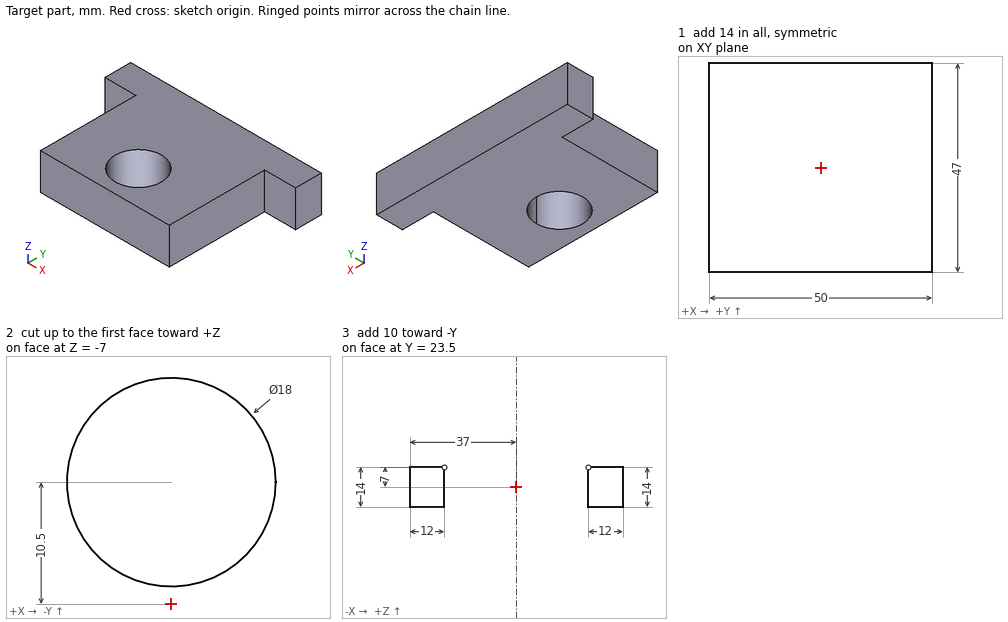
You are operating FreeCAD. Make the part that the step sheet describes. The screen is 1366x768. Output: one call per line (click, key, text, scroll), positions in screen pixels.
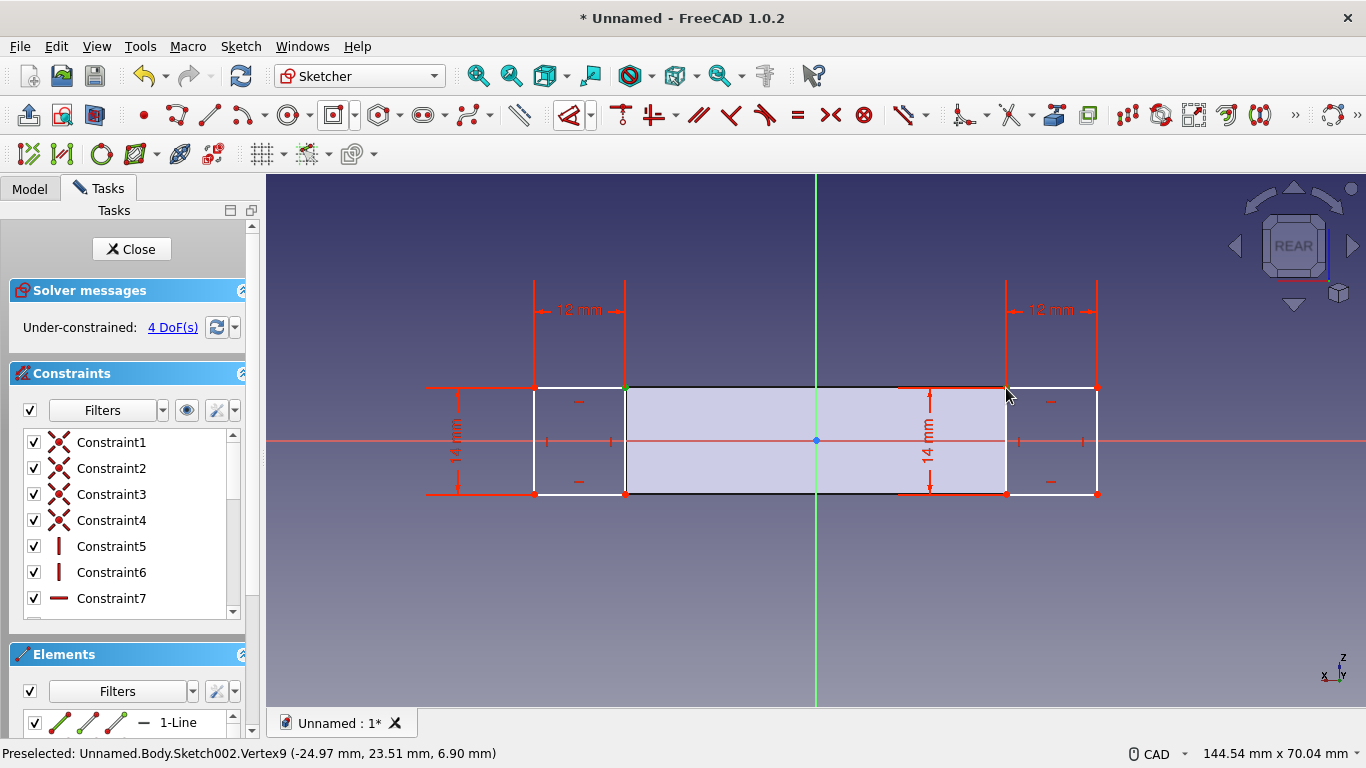
click(816, 645)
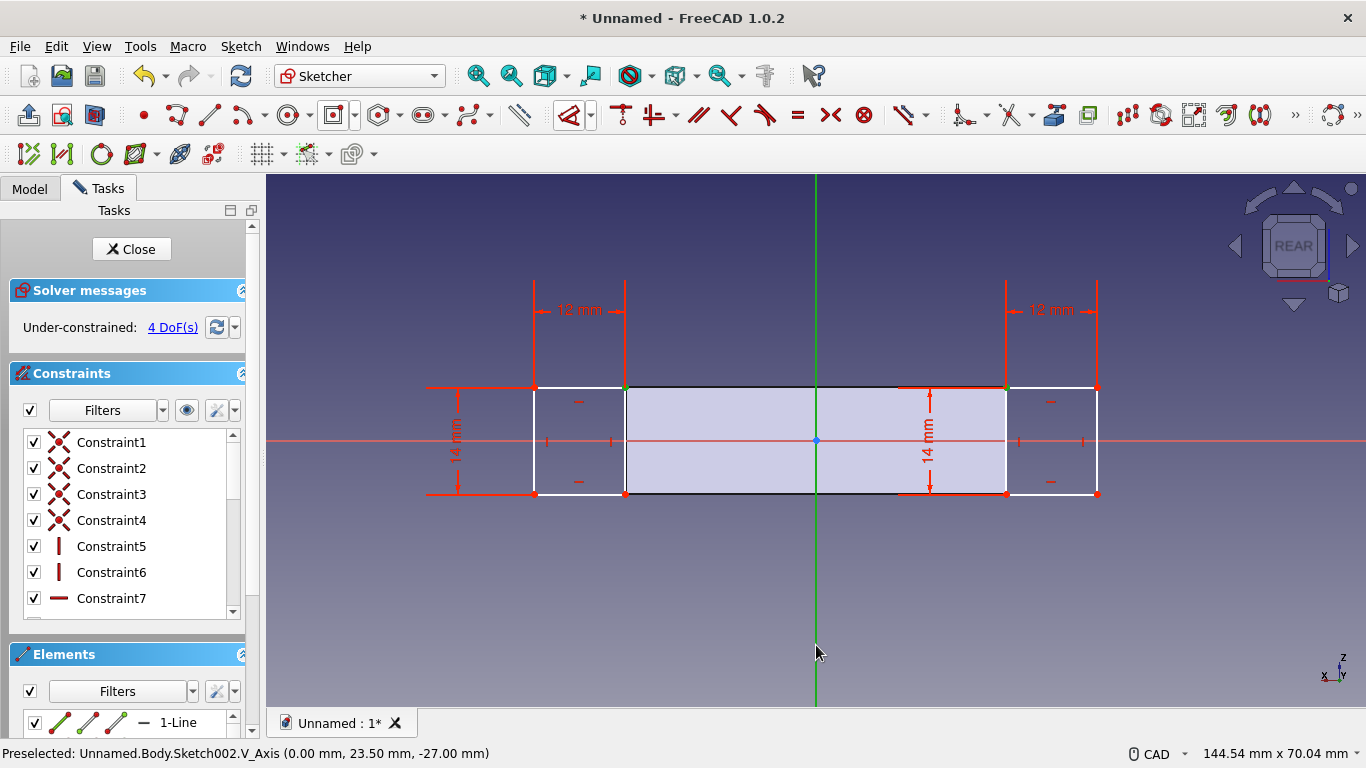
click(831, 116)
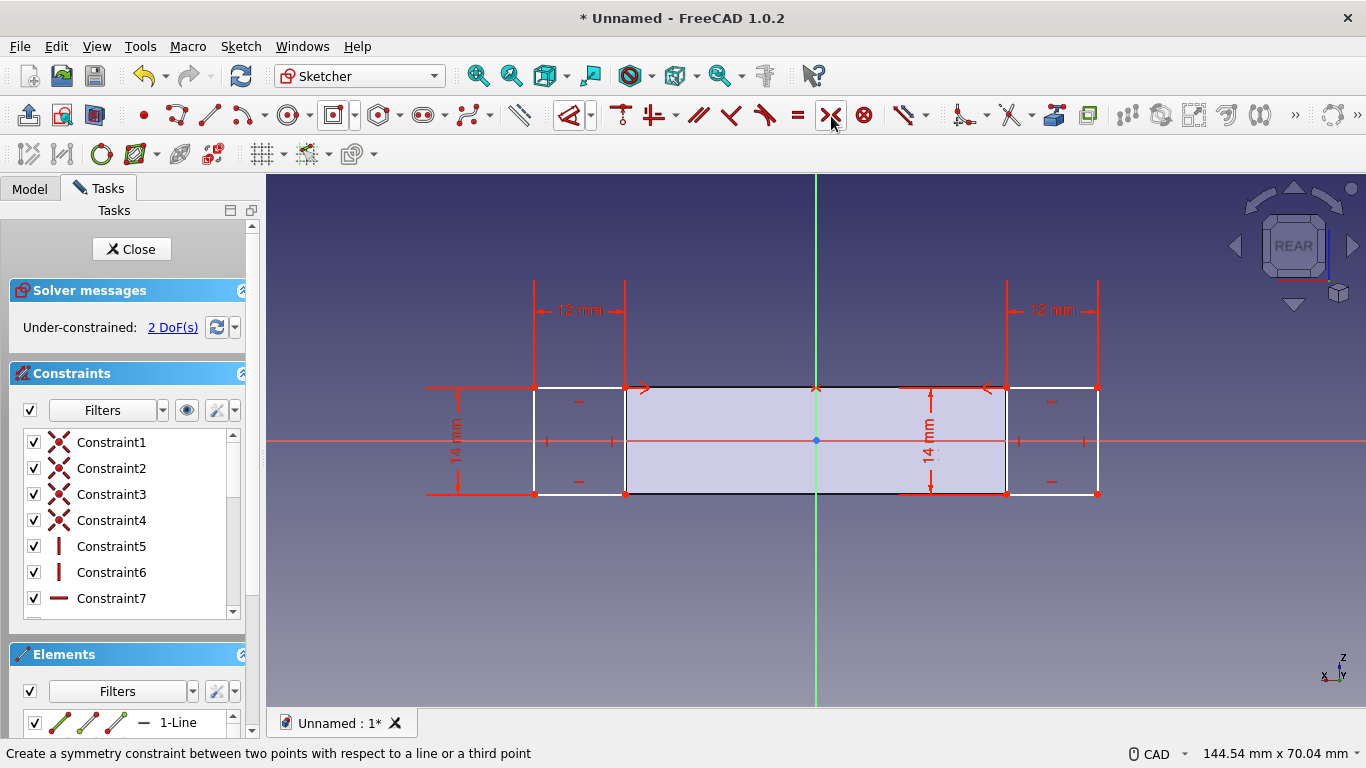
click(534, 388)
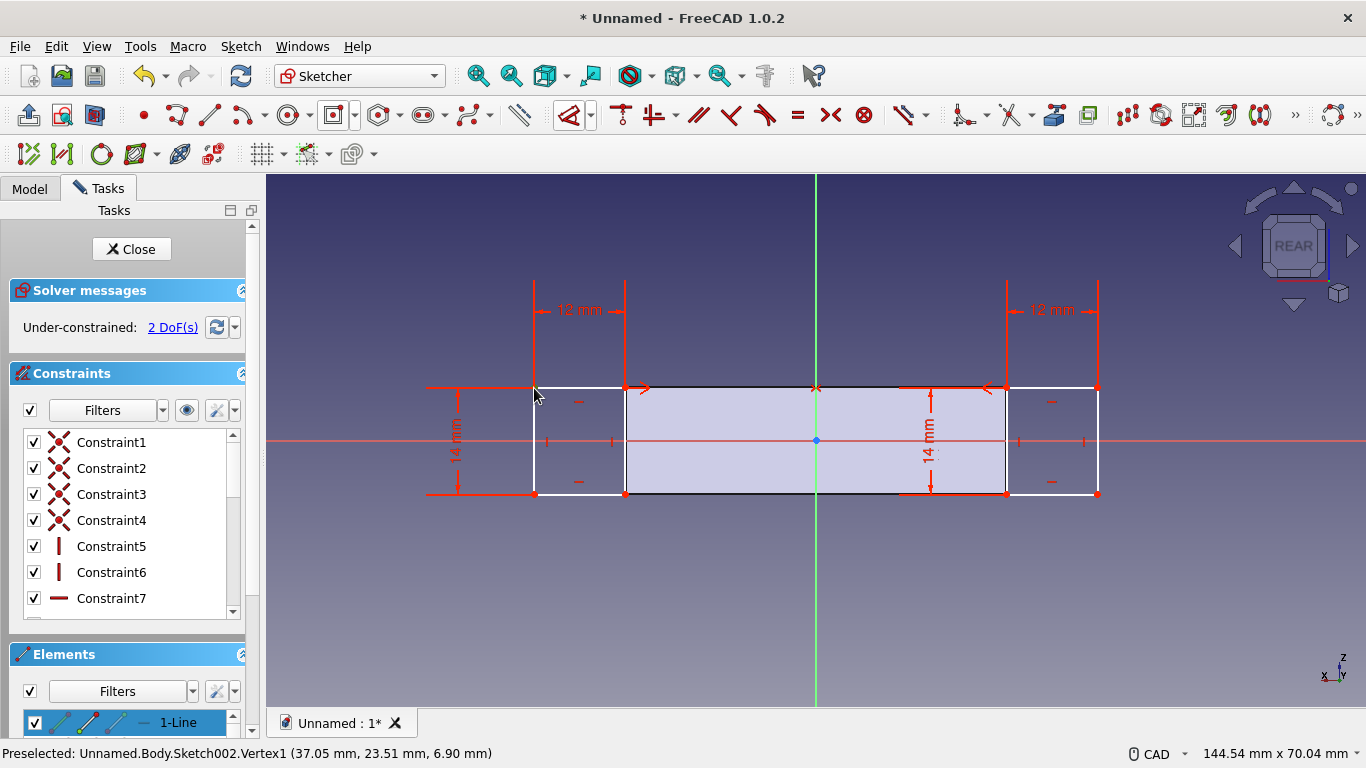
click(590, 116)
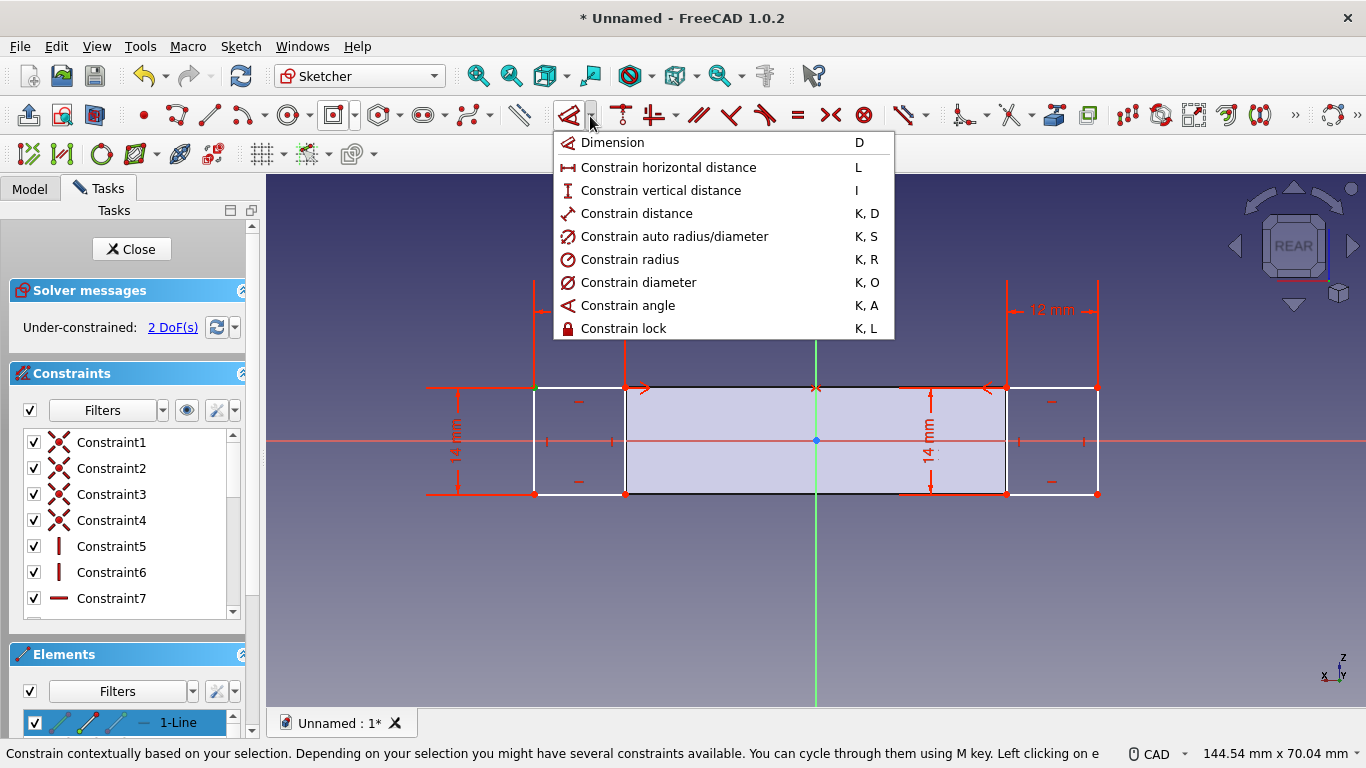
click(724, 190)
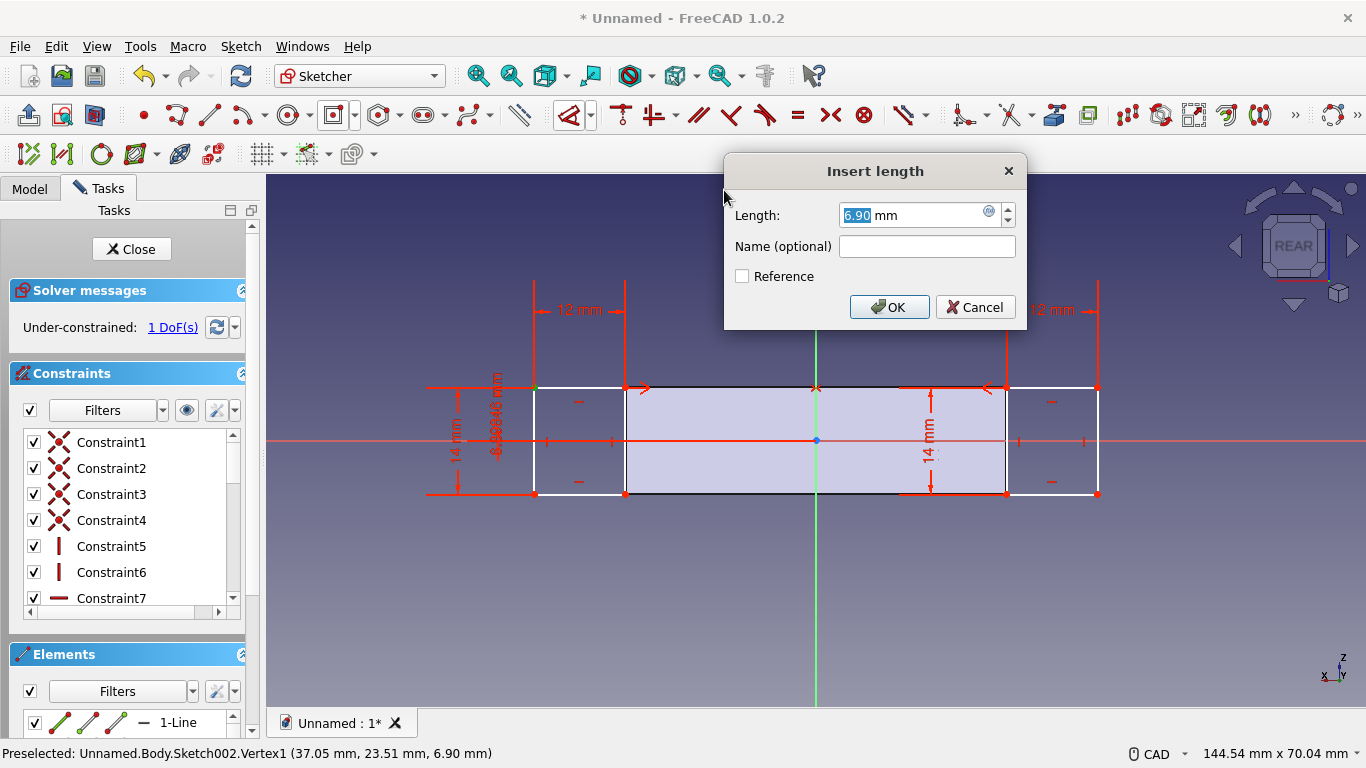
text(7)
key(Return)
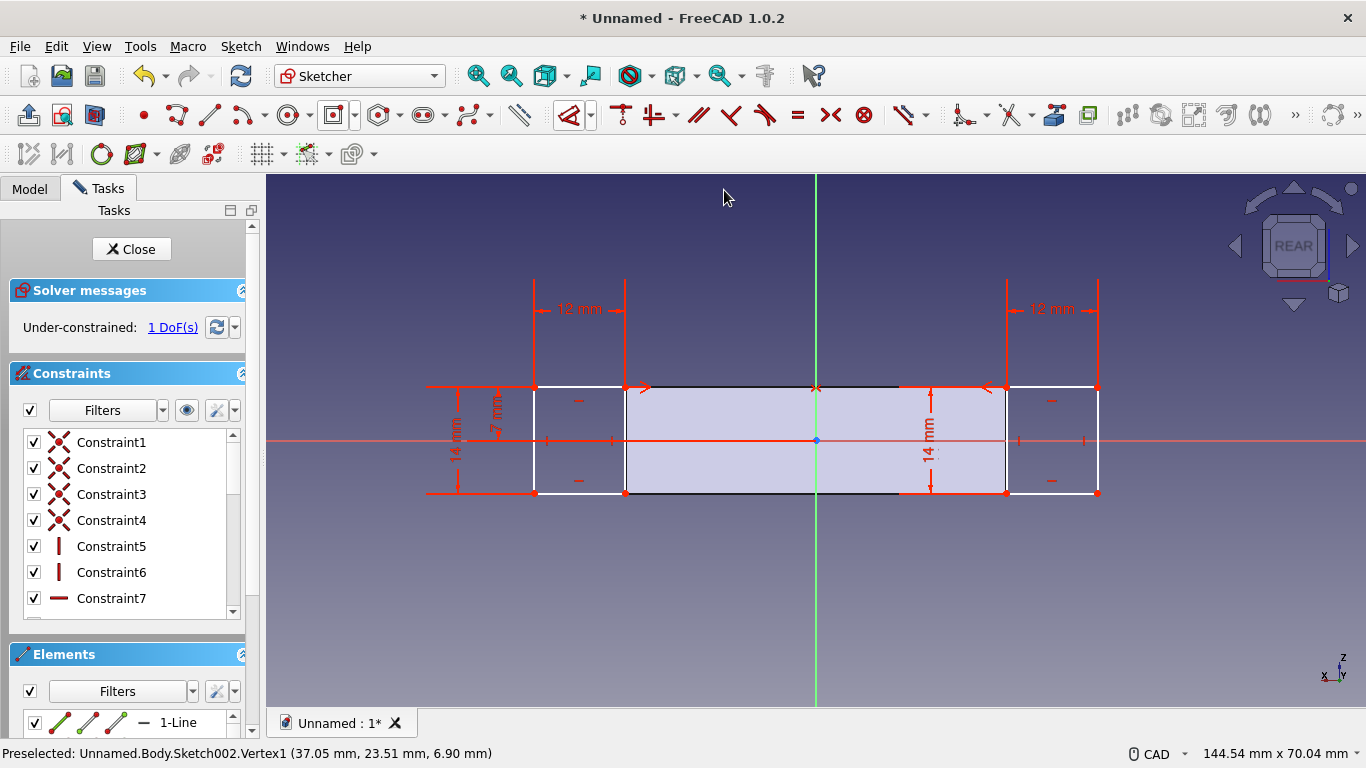
click(534, 387)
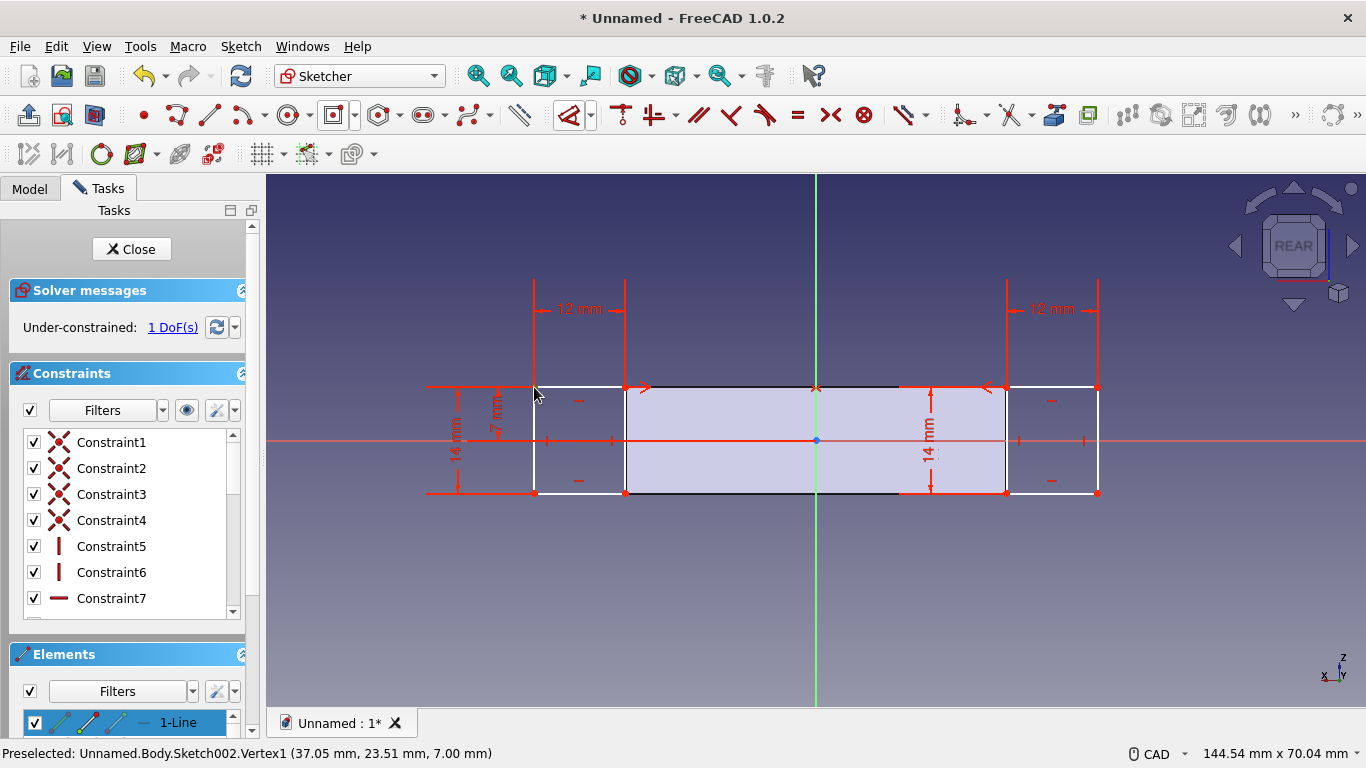
key(l)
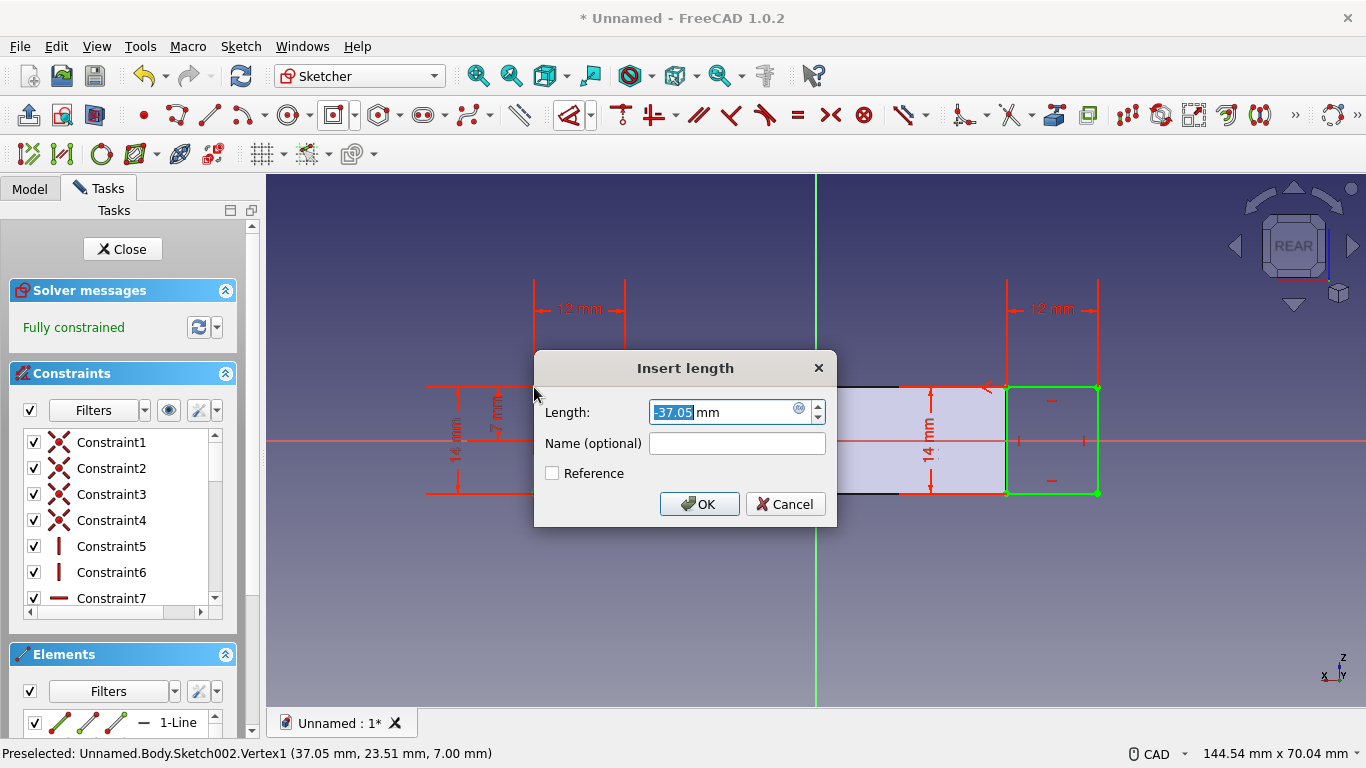
text(-37)
key(Return)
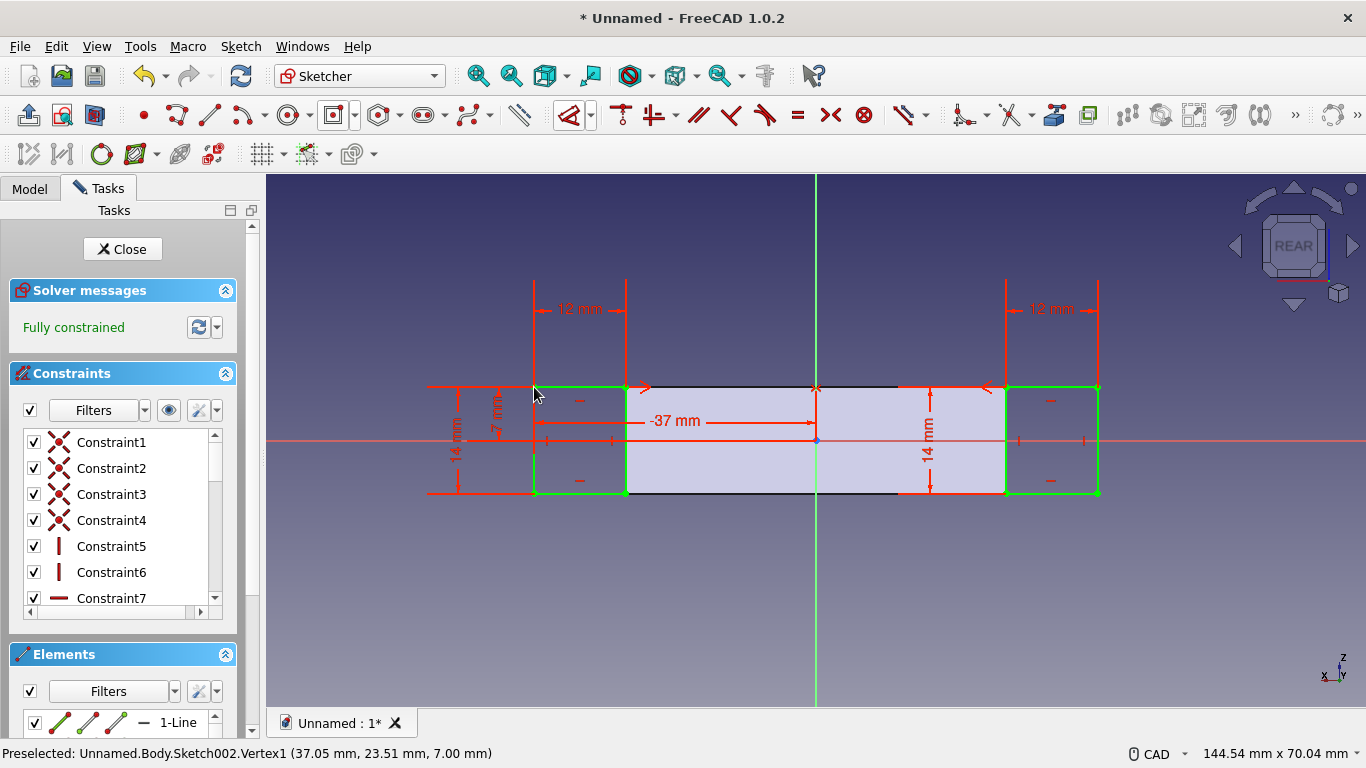
click(123, 249)